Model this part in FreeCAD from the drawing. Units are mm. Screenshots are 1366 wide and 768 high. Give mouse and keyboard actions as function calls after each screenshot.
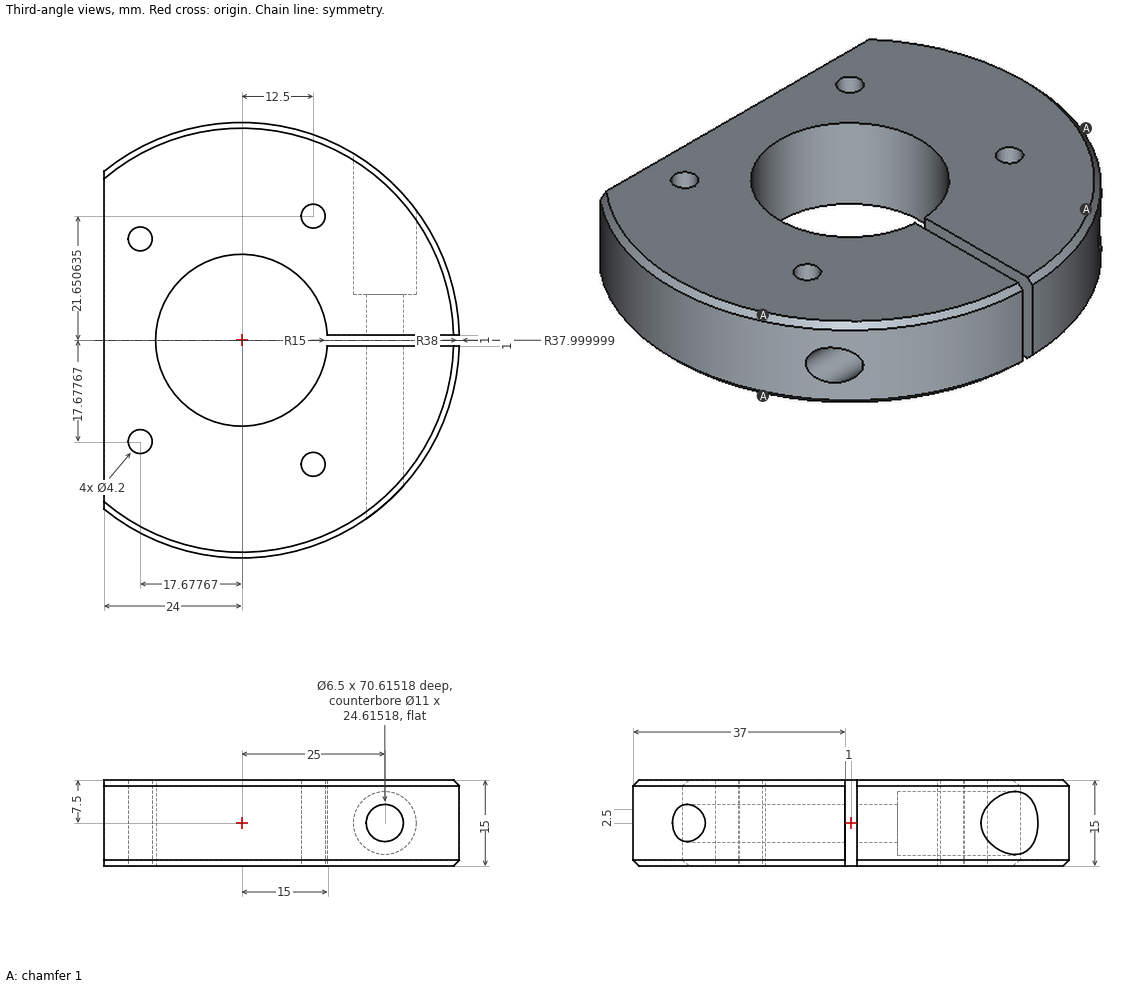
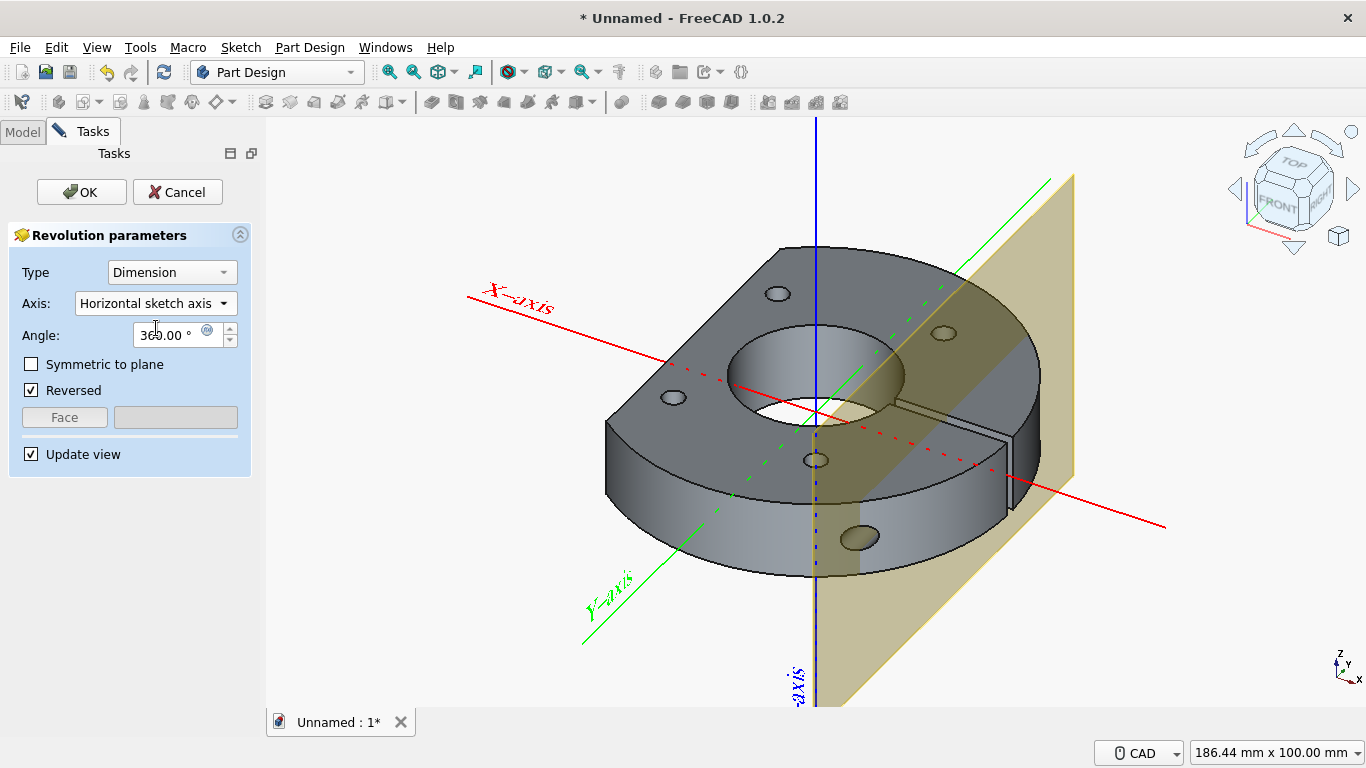
click(82, 192)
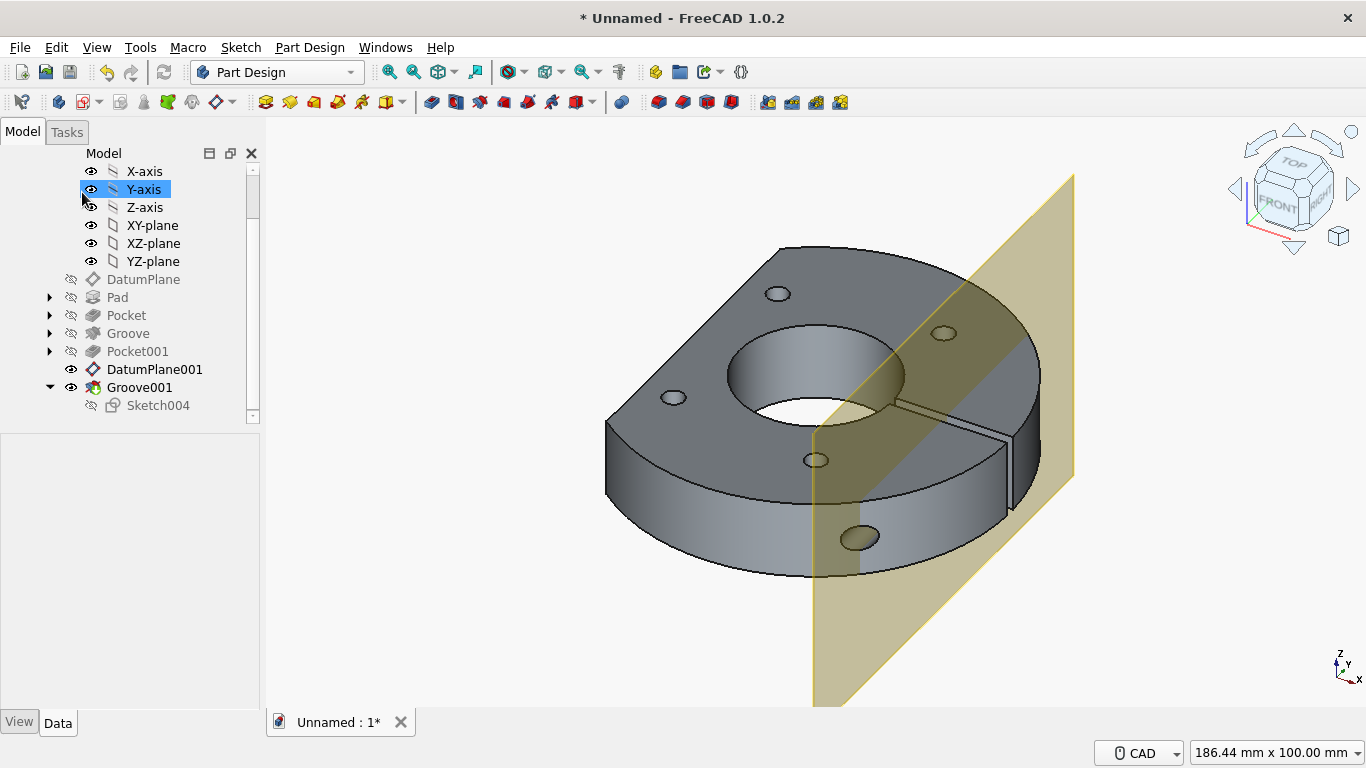
click(116, 369)
key(space)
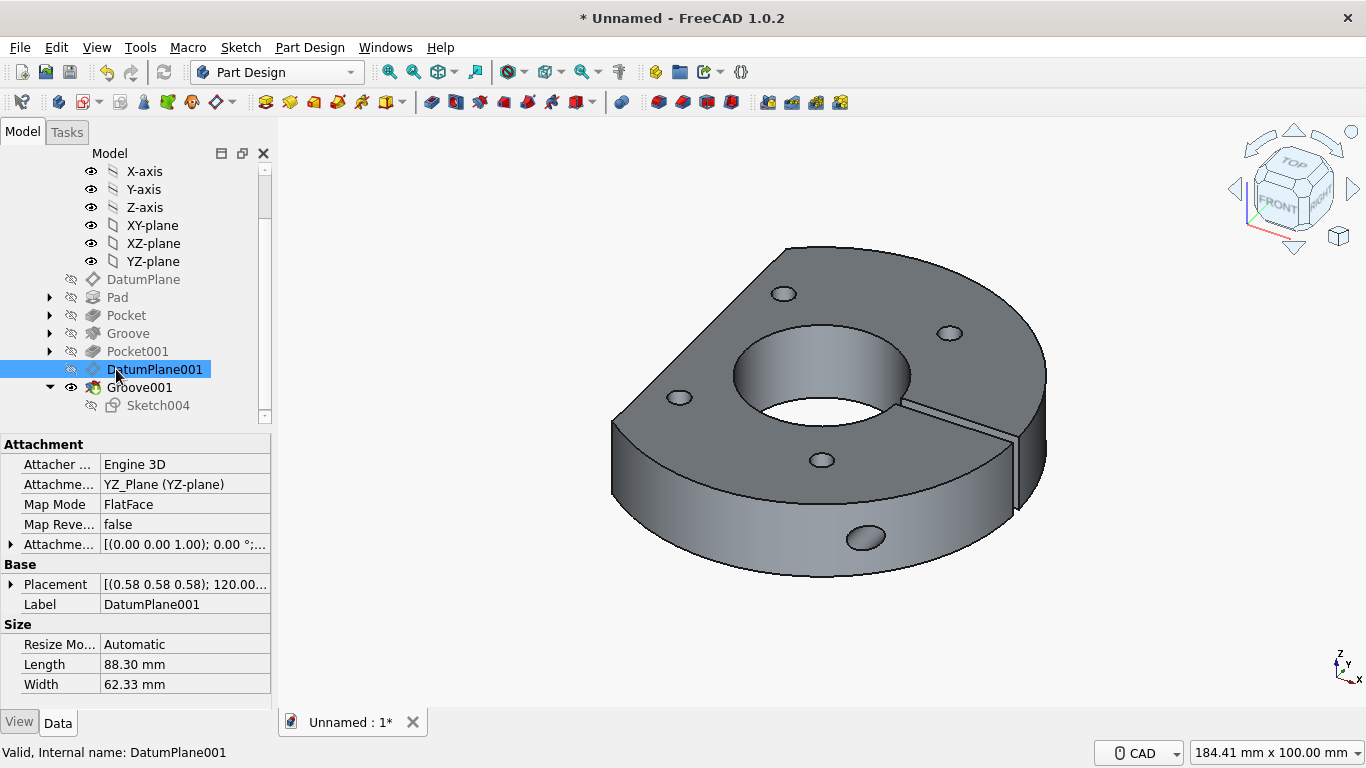
scroll(160, 293, down, 3)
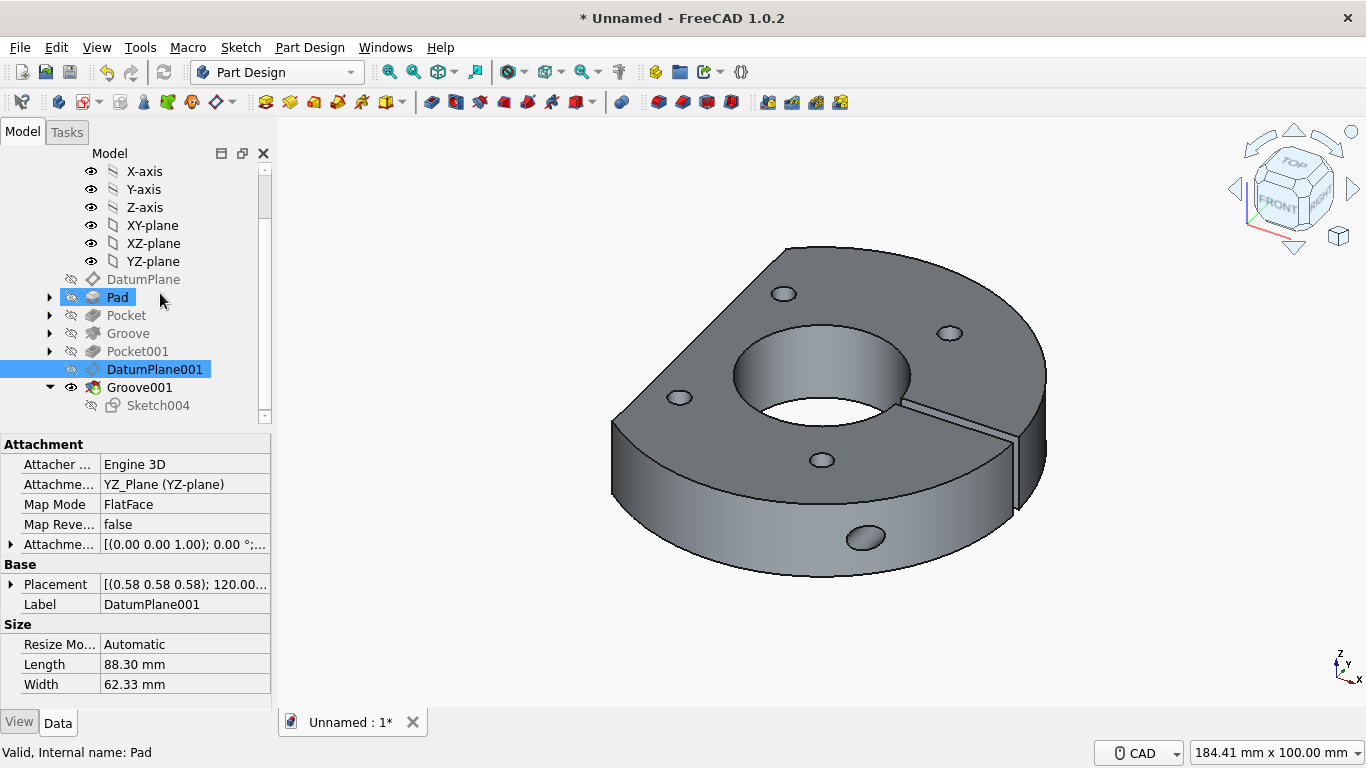
scroll(160, 293, up, 15)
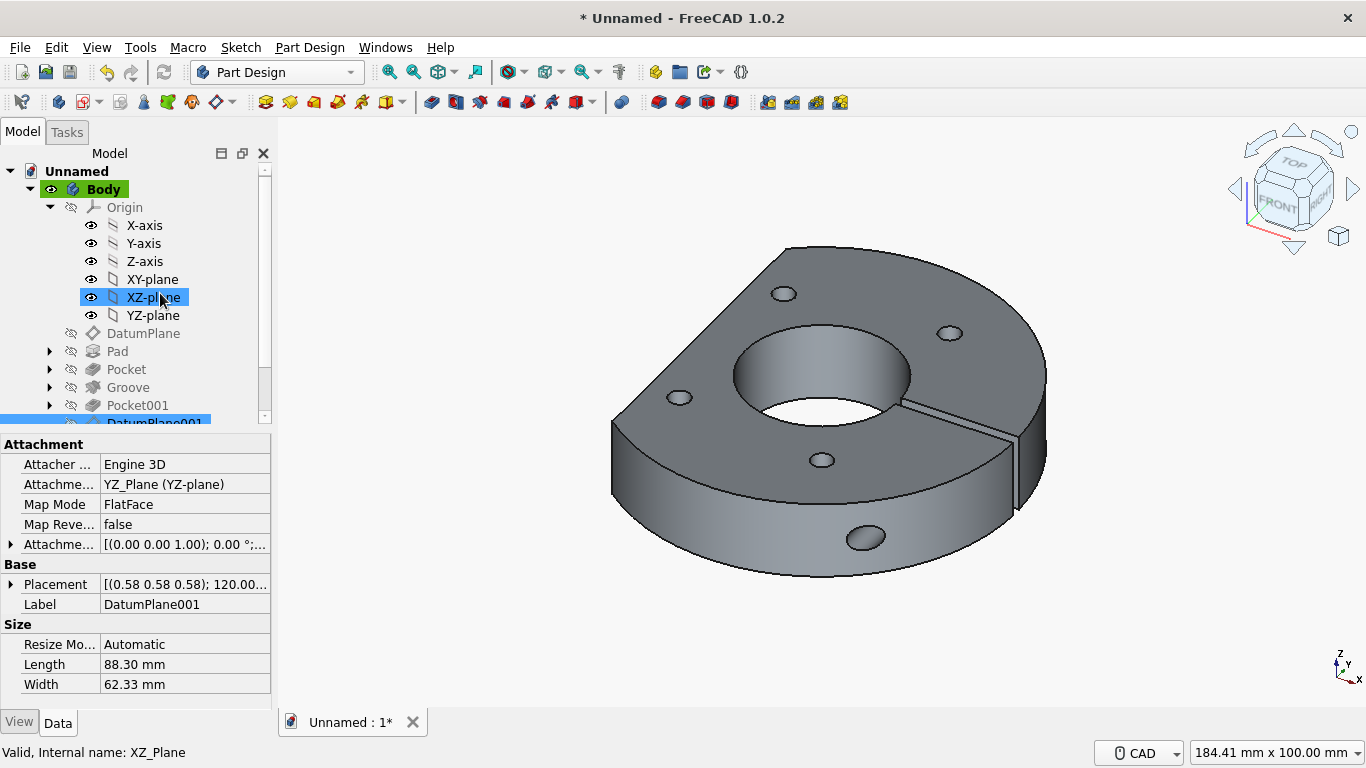
click(136, 297)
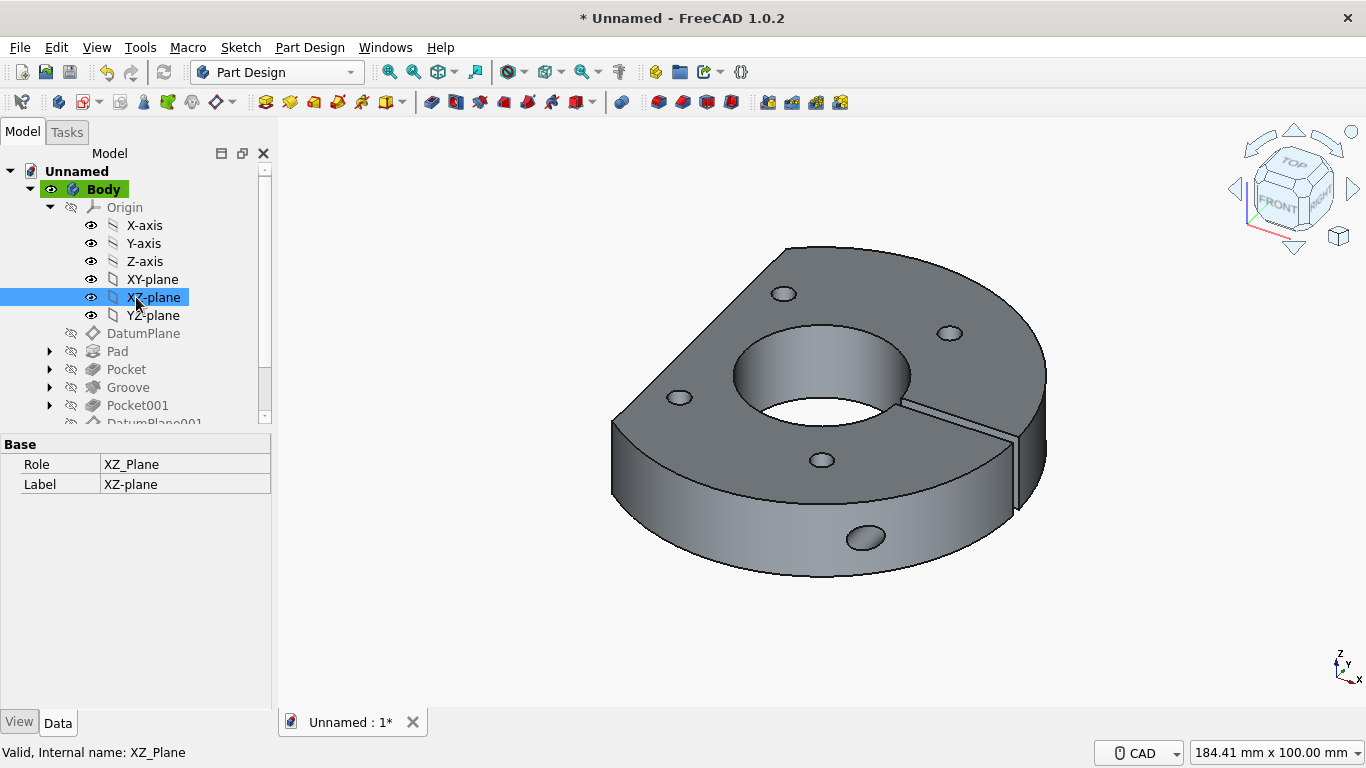
click(216, 102)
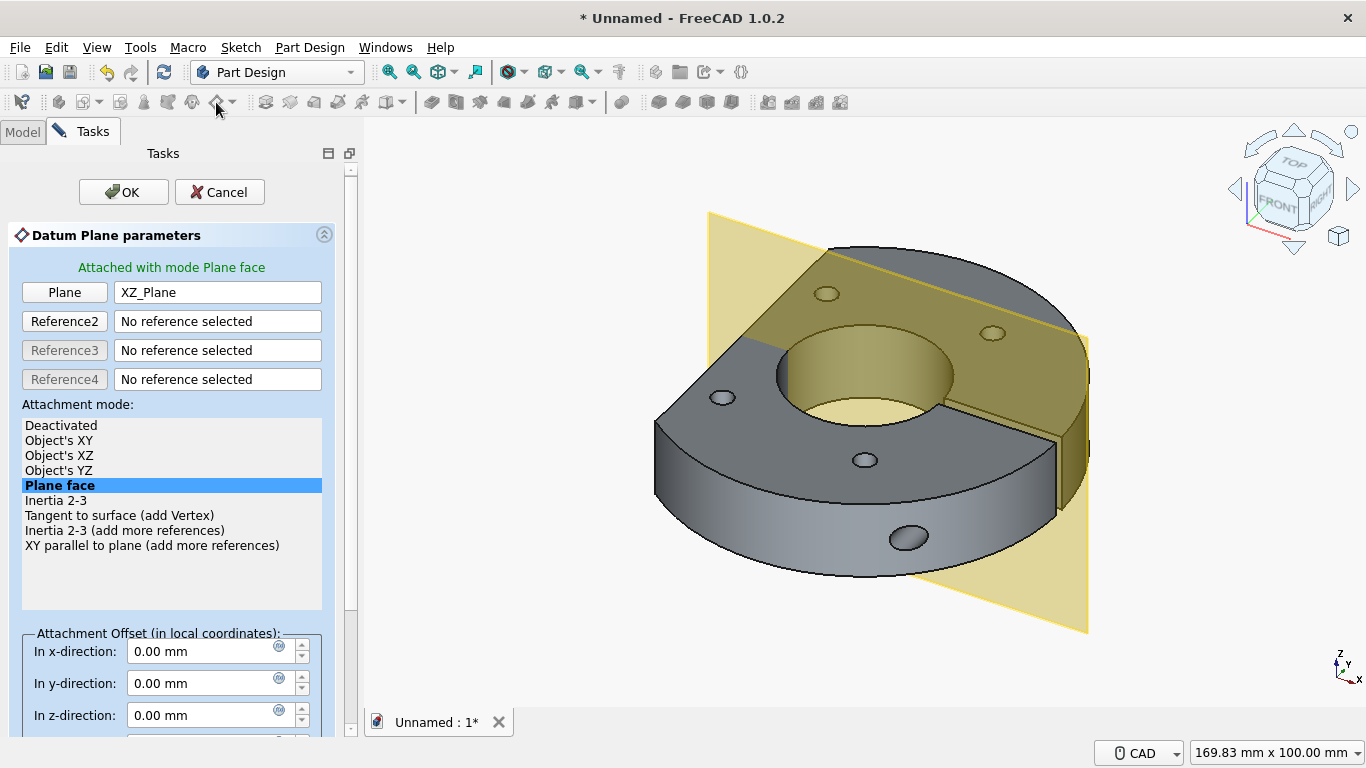
triple_click(210, 715)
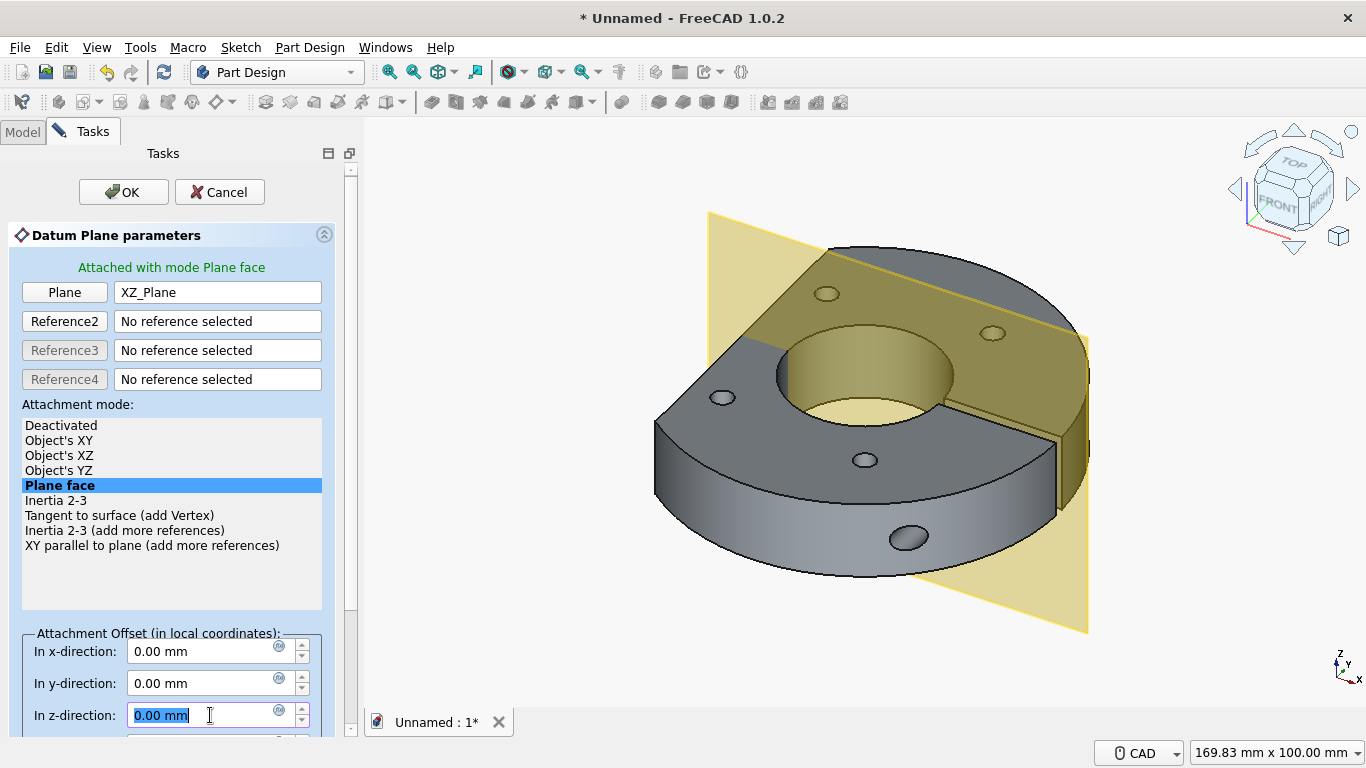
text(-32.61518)
key(Tab)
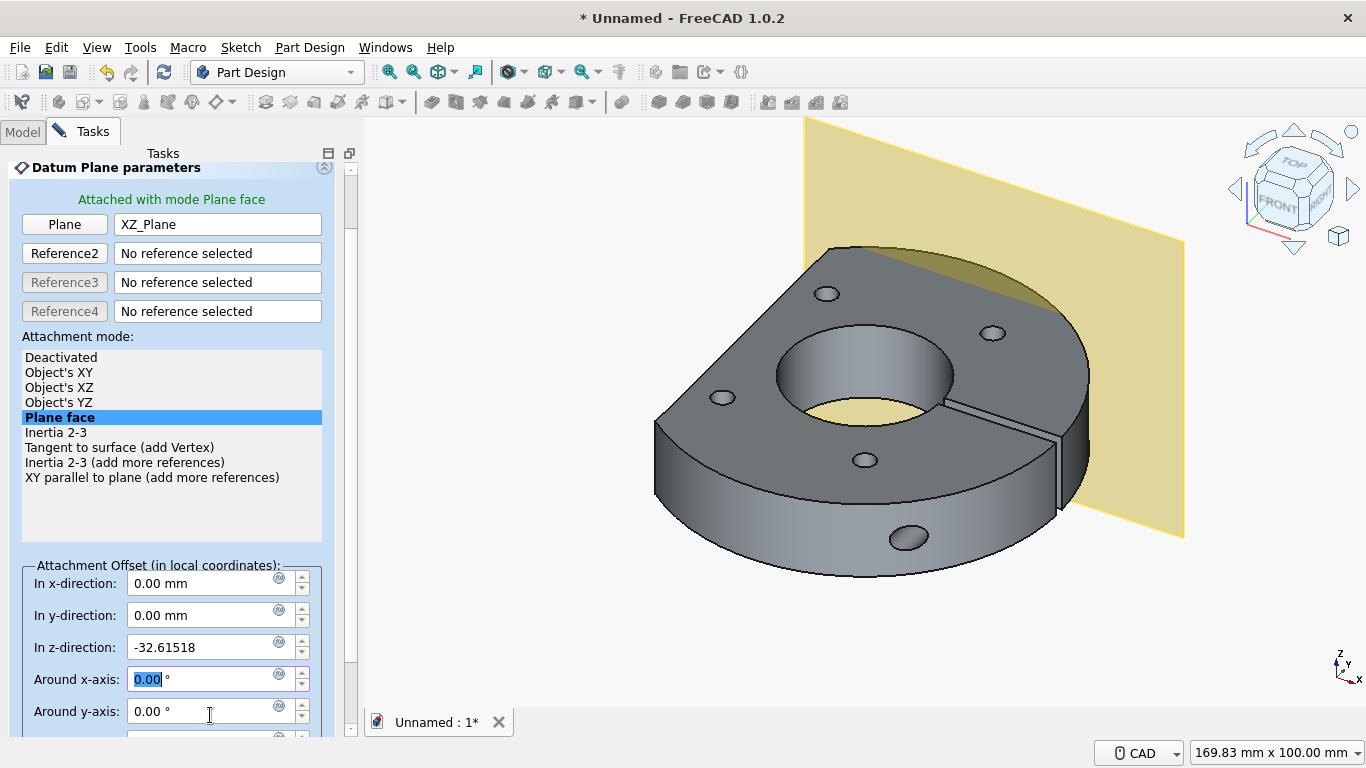
scroll(351, 450, up, 2)